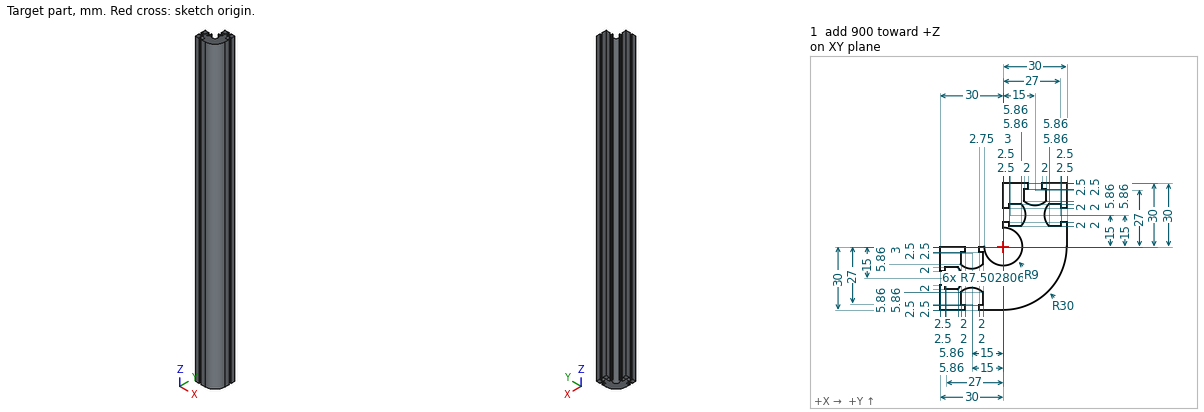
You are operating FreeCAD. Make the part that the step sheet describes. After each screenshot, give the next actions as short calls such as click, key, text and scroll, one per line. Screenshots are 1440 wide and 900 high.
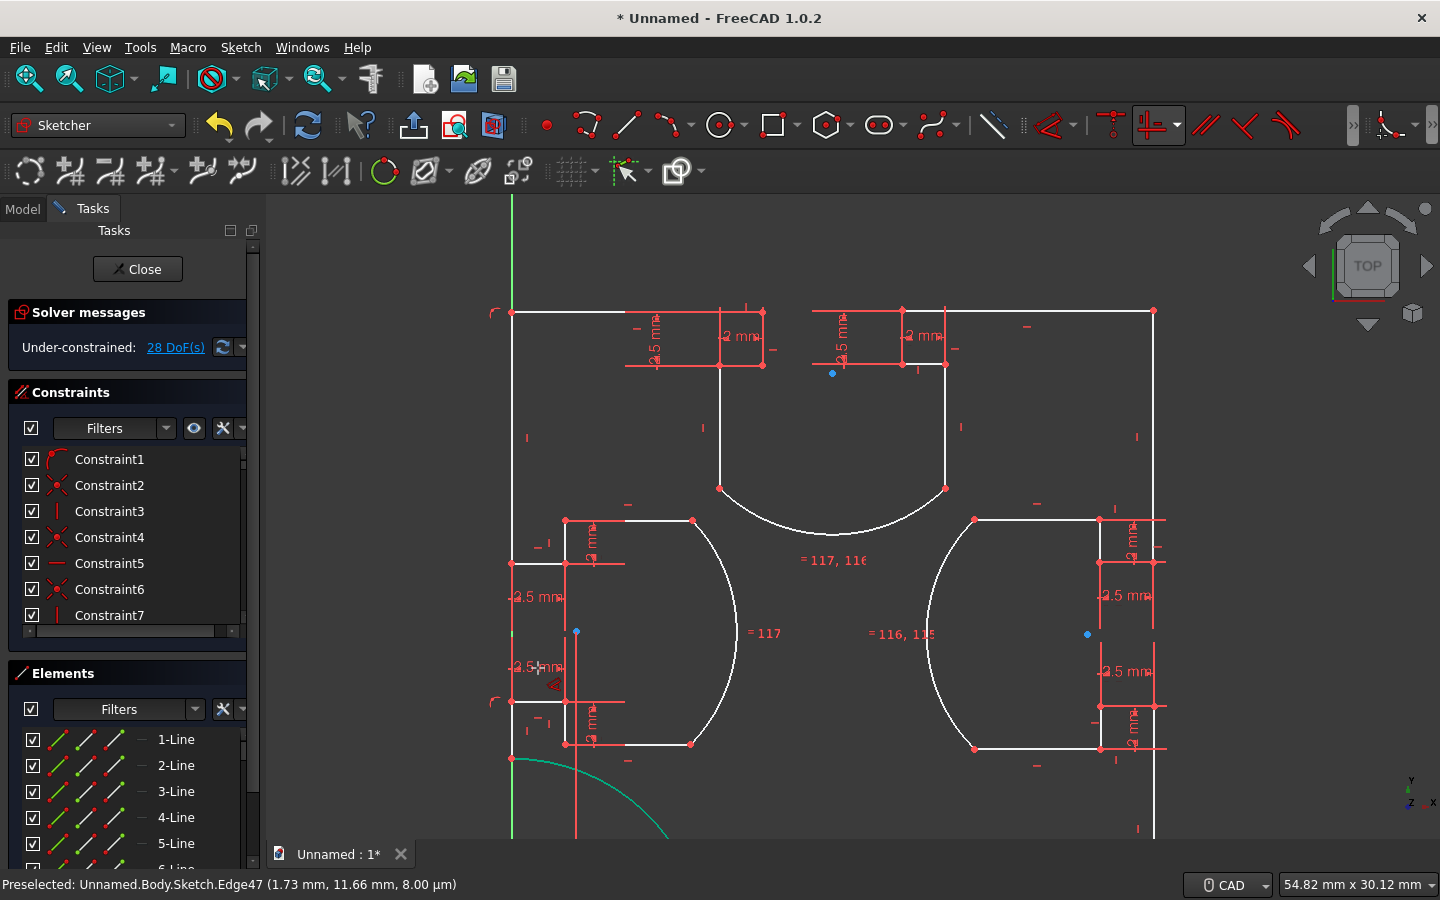
scroll(902, 329, down, 6)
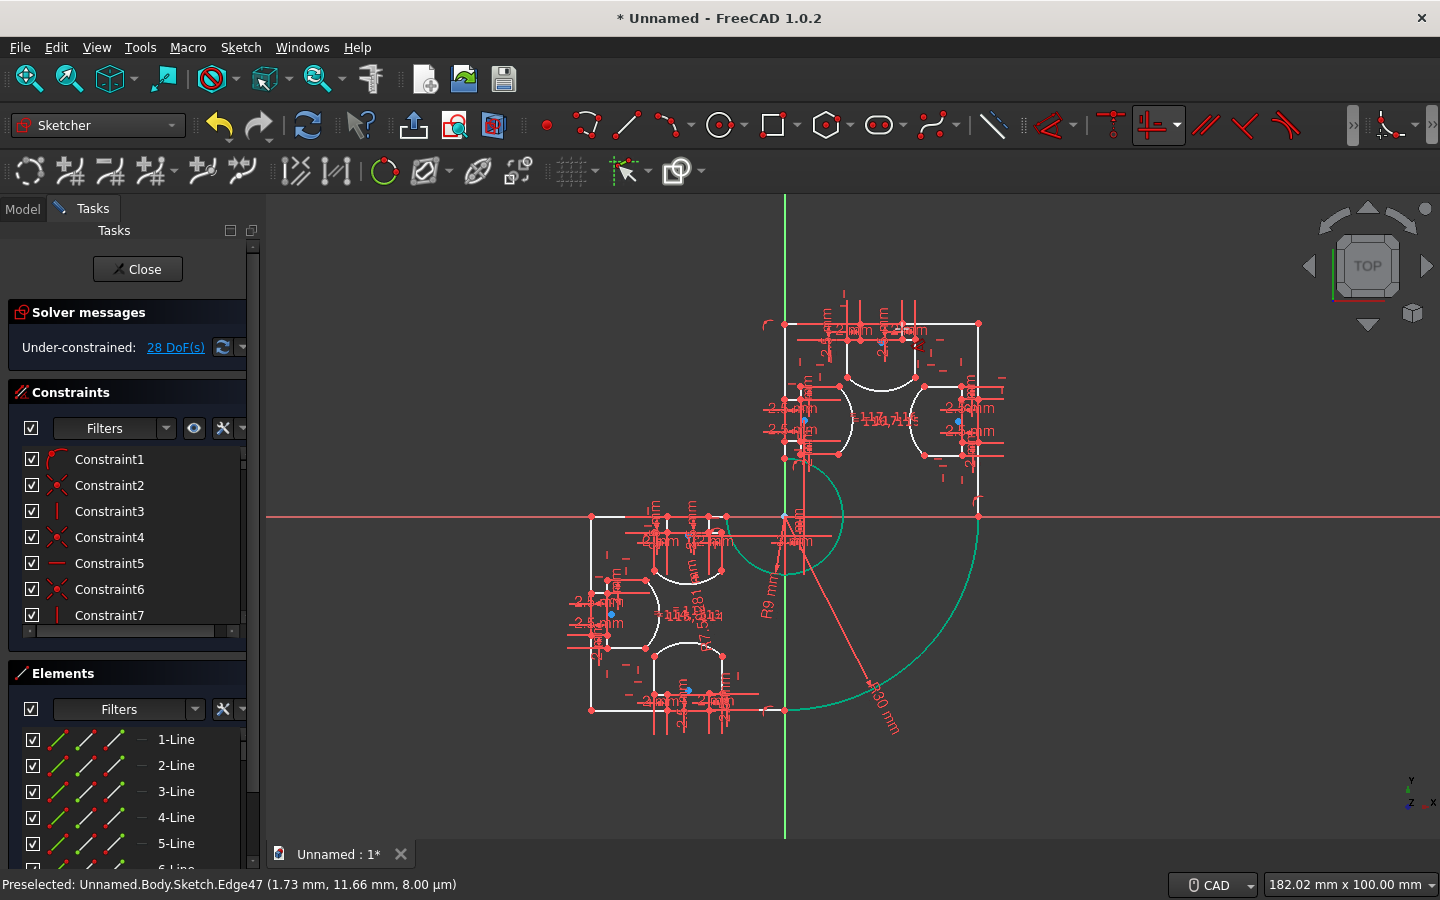
click(591, 517)
click(688, 483)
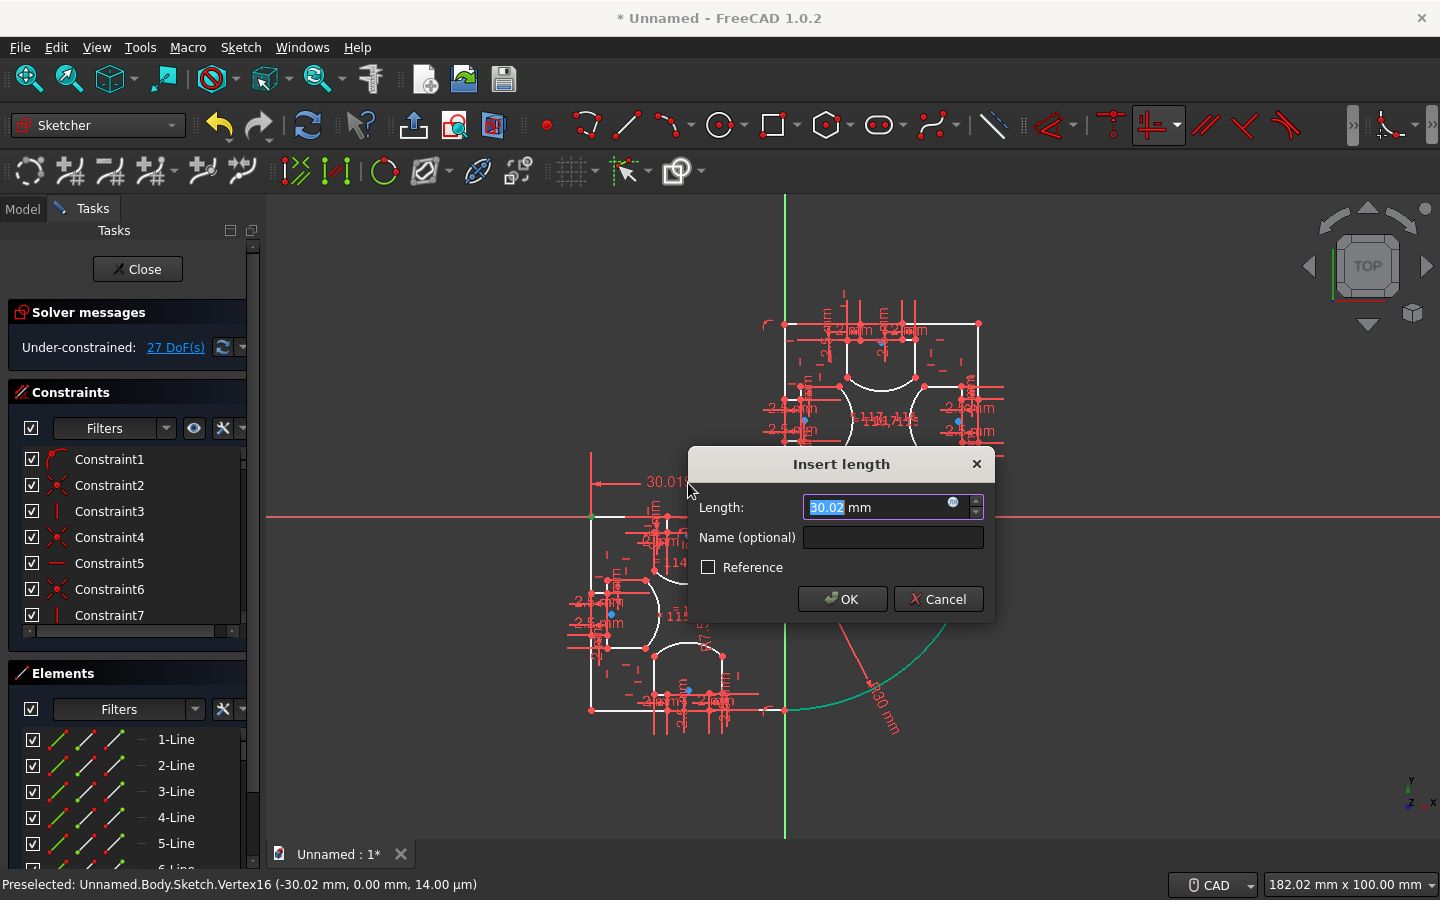
text(30)
key(Return)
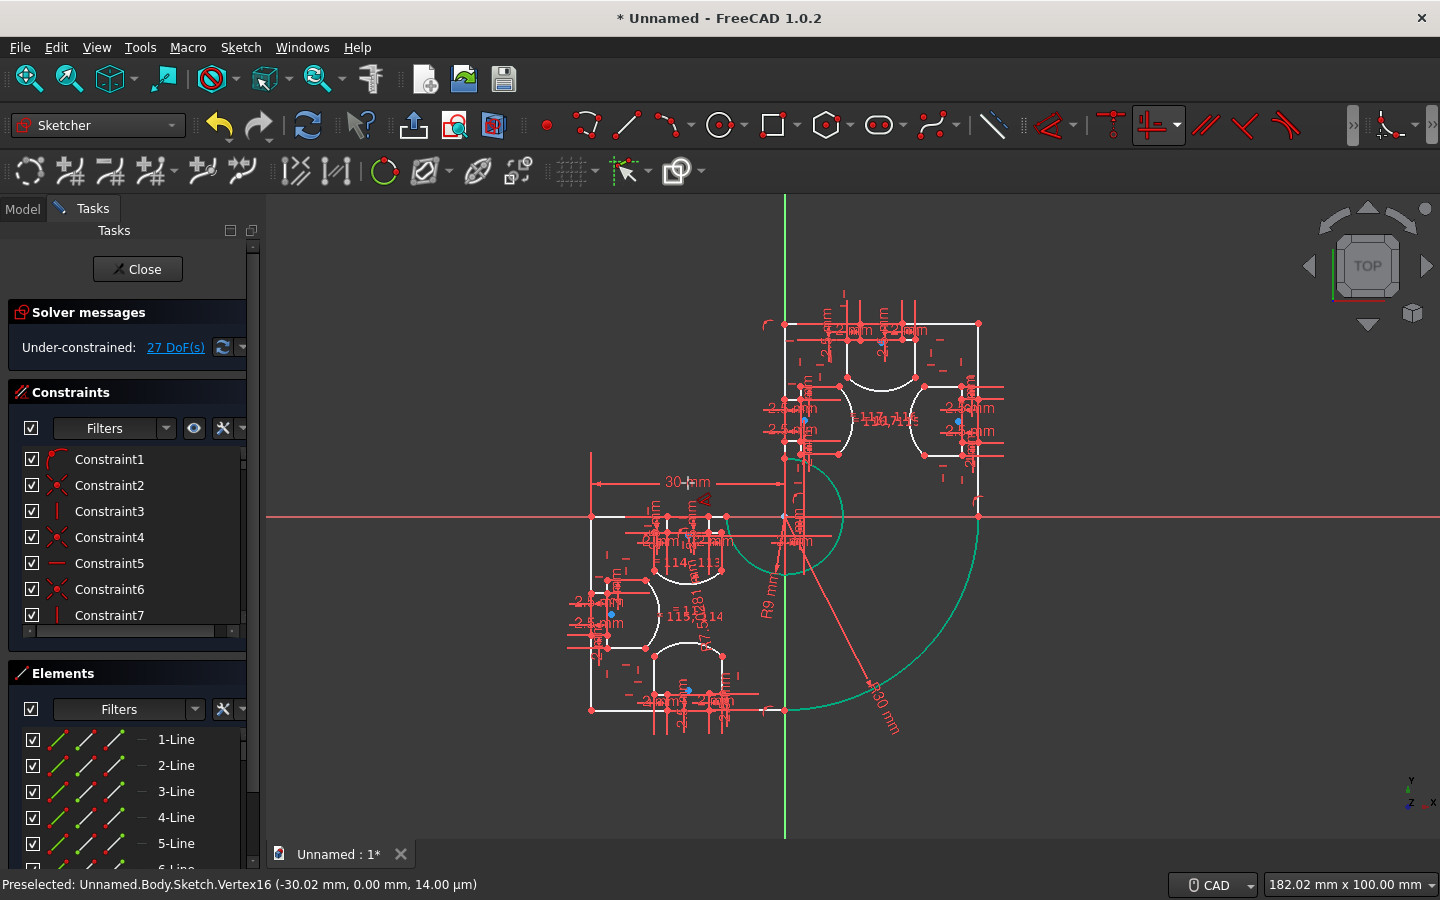
click(591, 635)
click(688, 669)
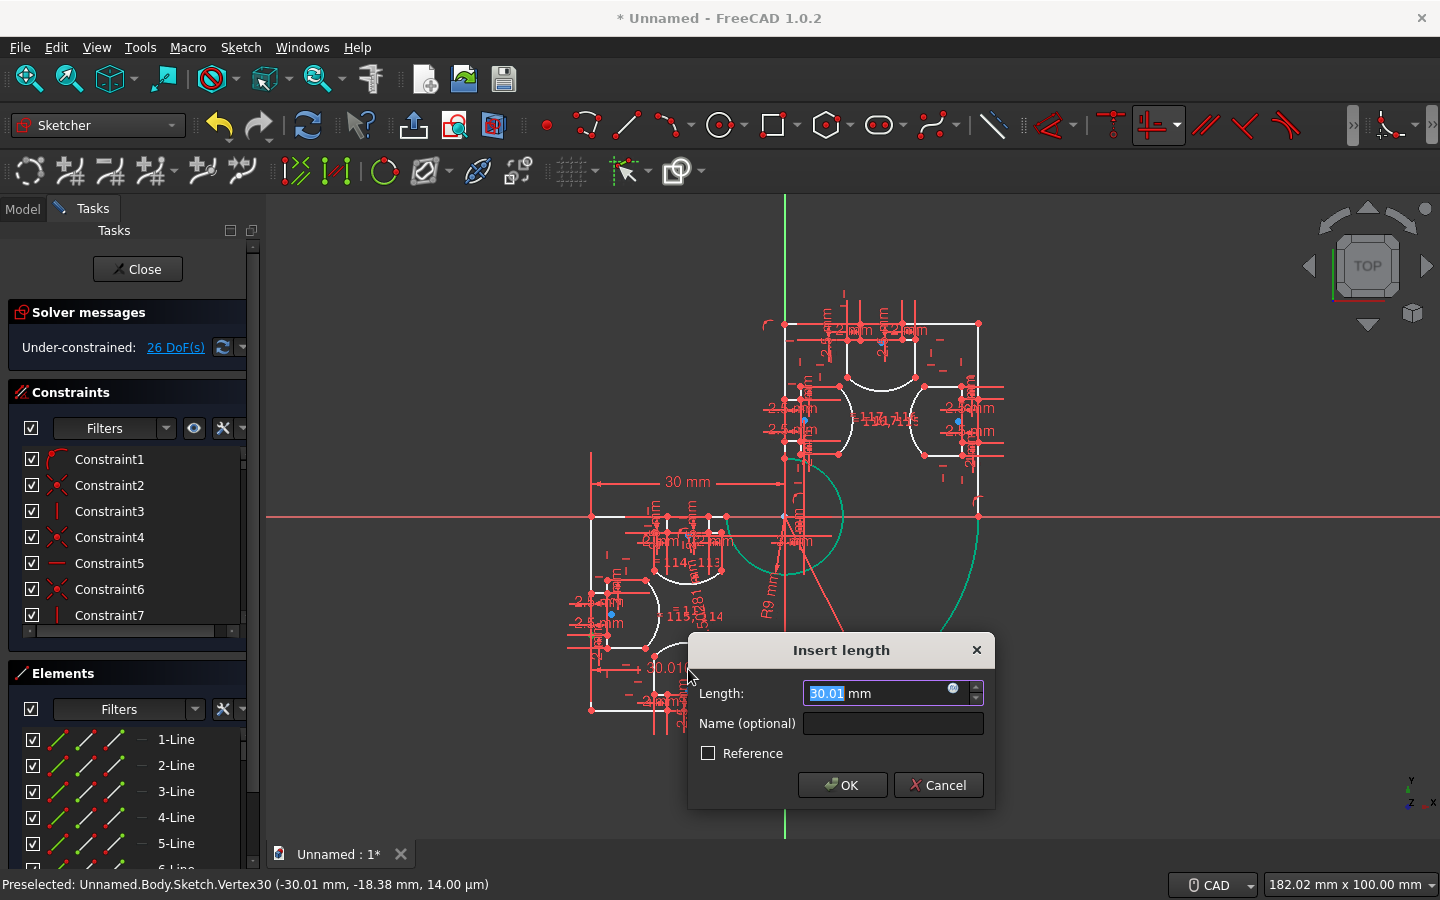
text(30)
key(Return)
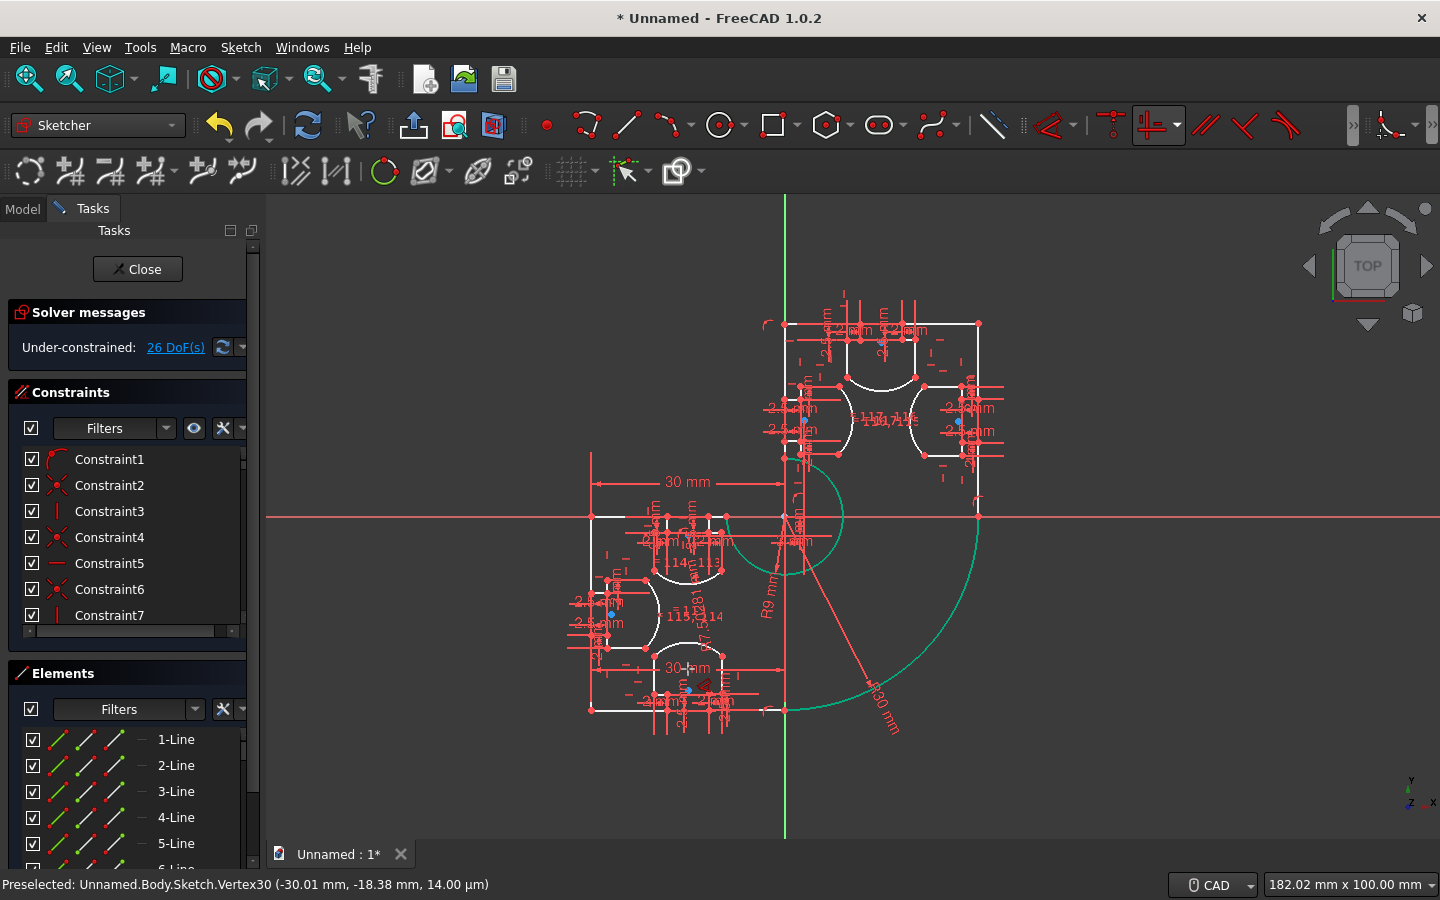
click(591, 711)
click(557, 546)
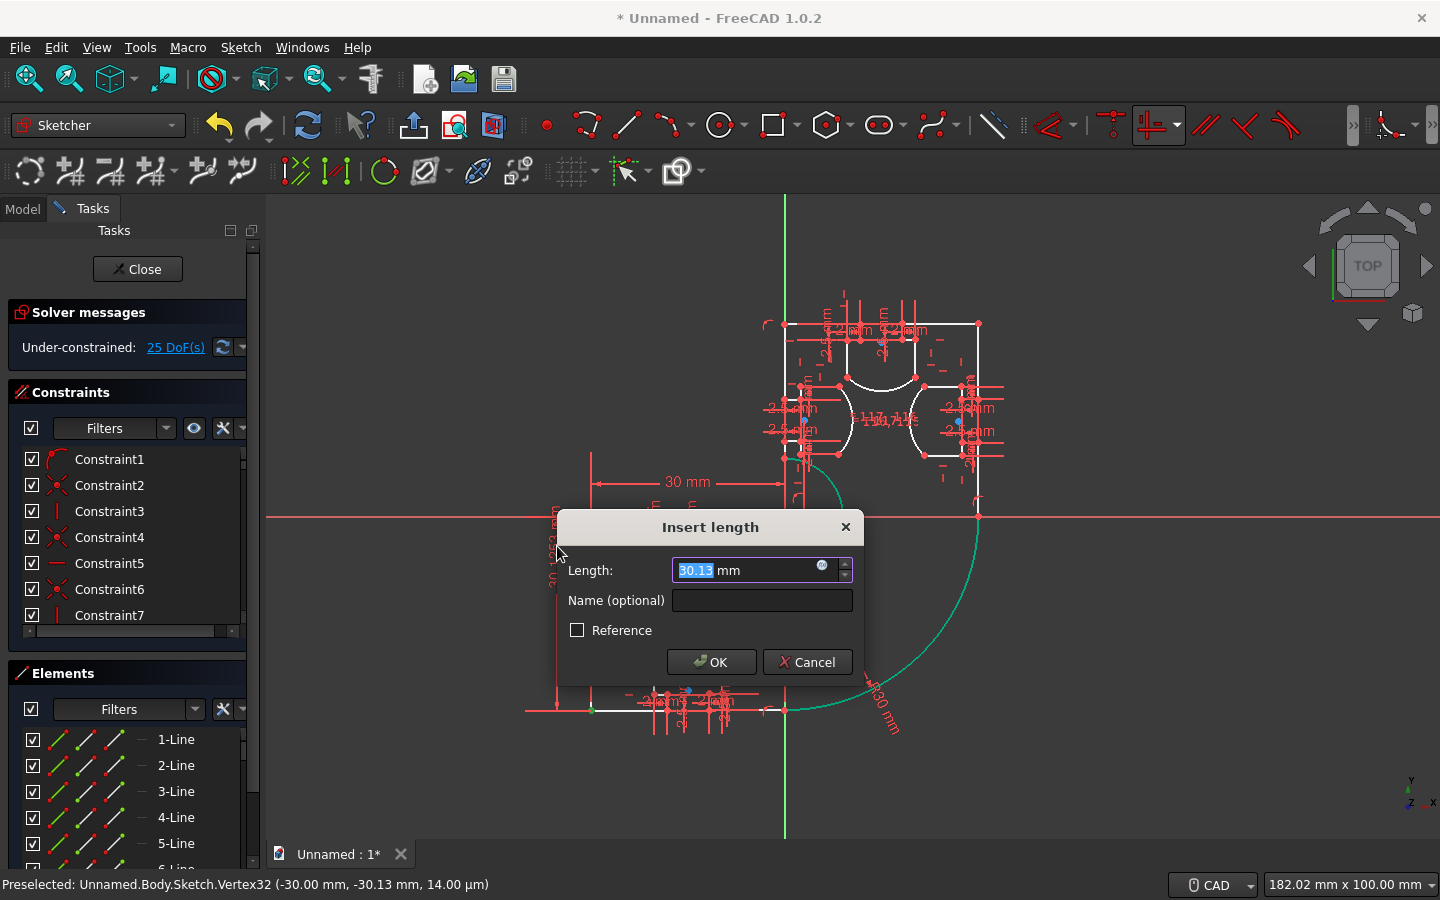
text(30)
key(Return)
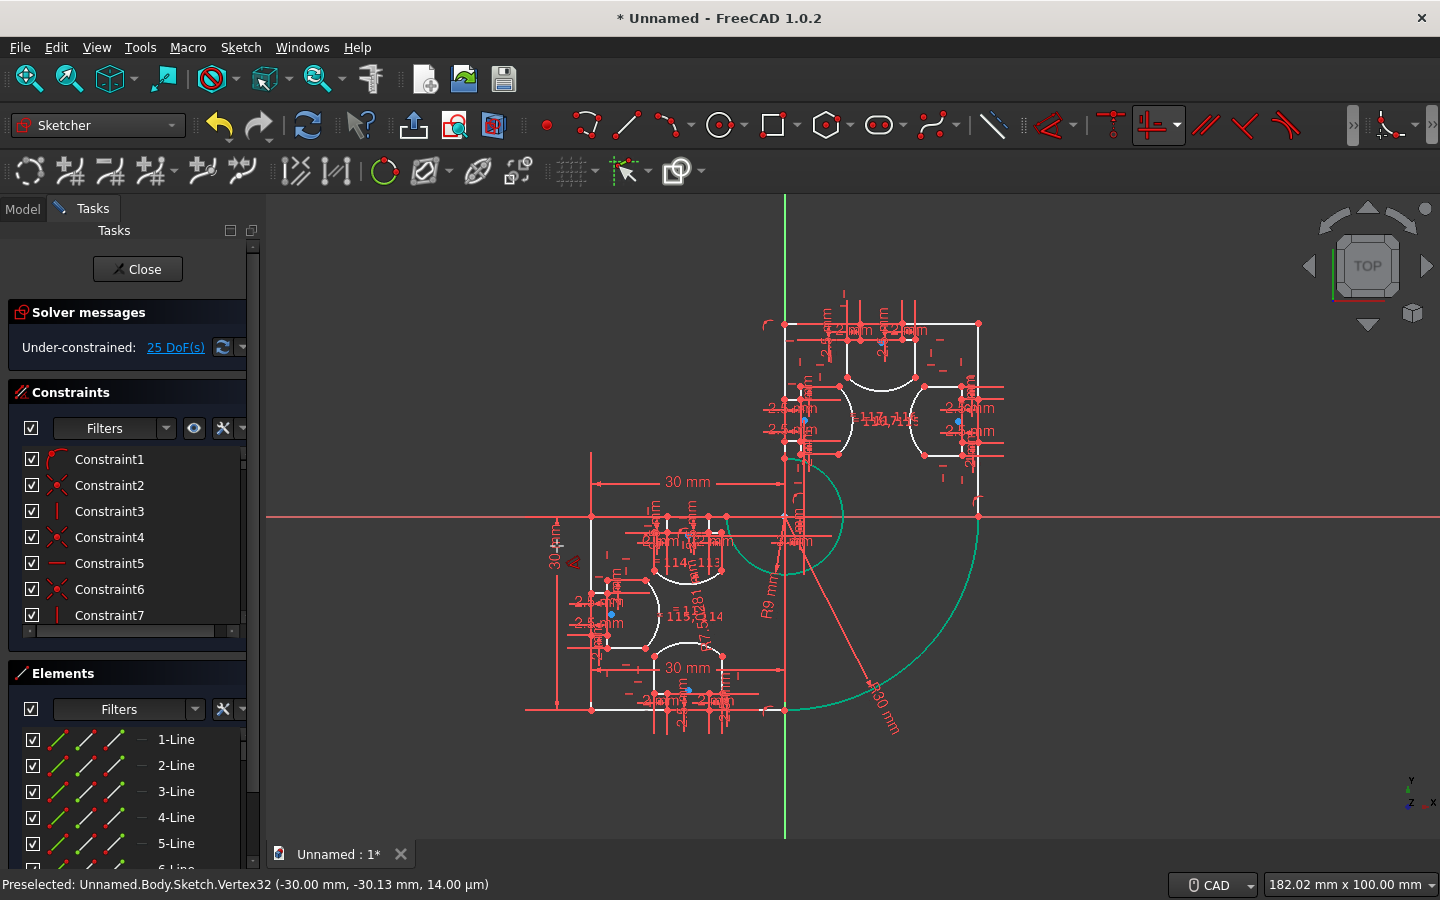
click(978, 399)
click(881, 365)